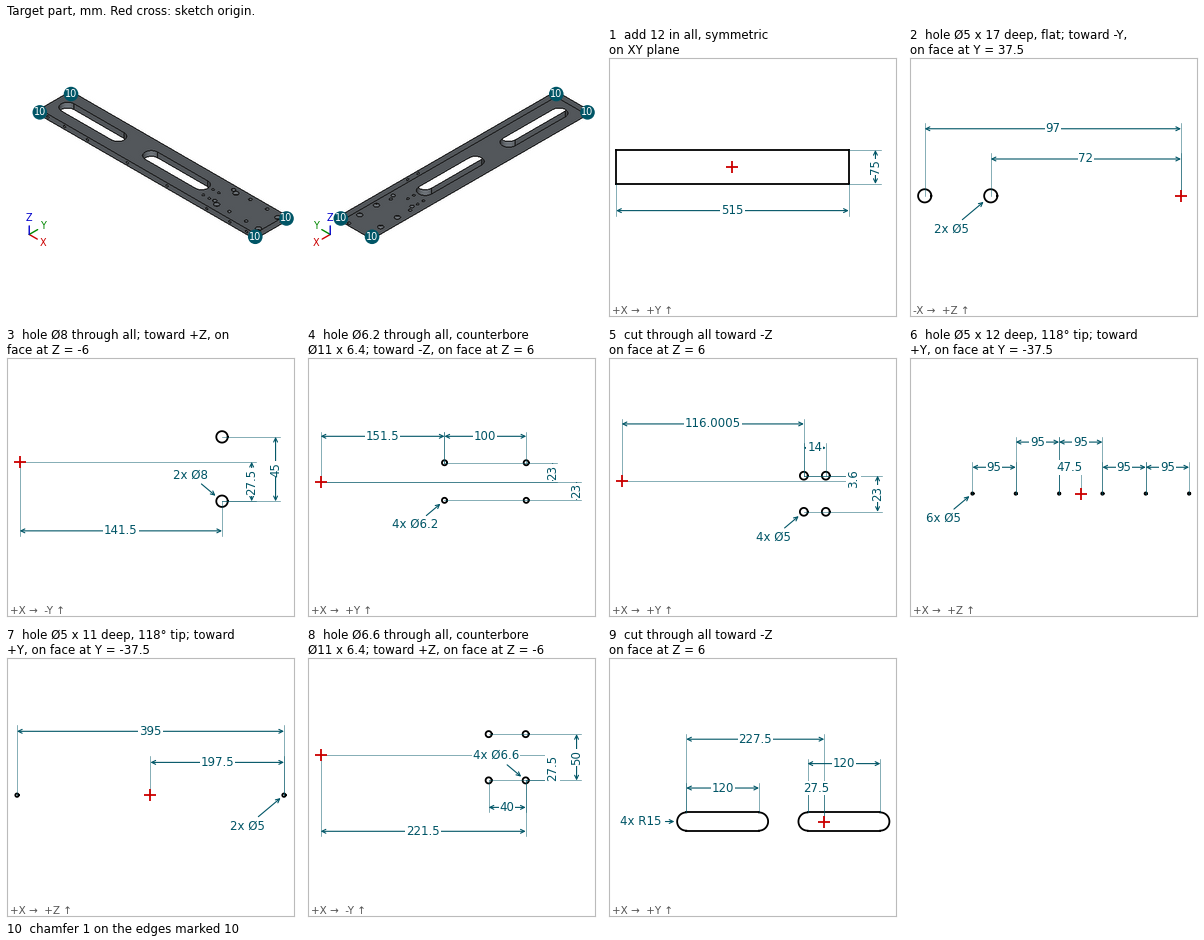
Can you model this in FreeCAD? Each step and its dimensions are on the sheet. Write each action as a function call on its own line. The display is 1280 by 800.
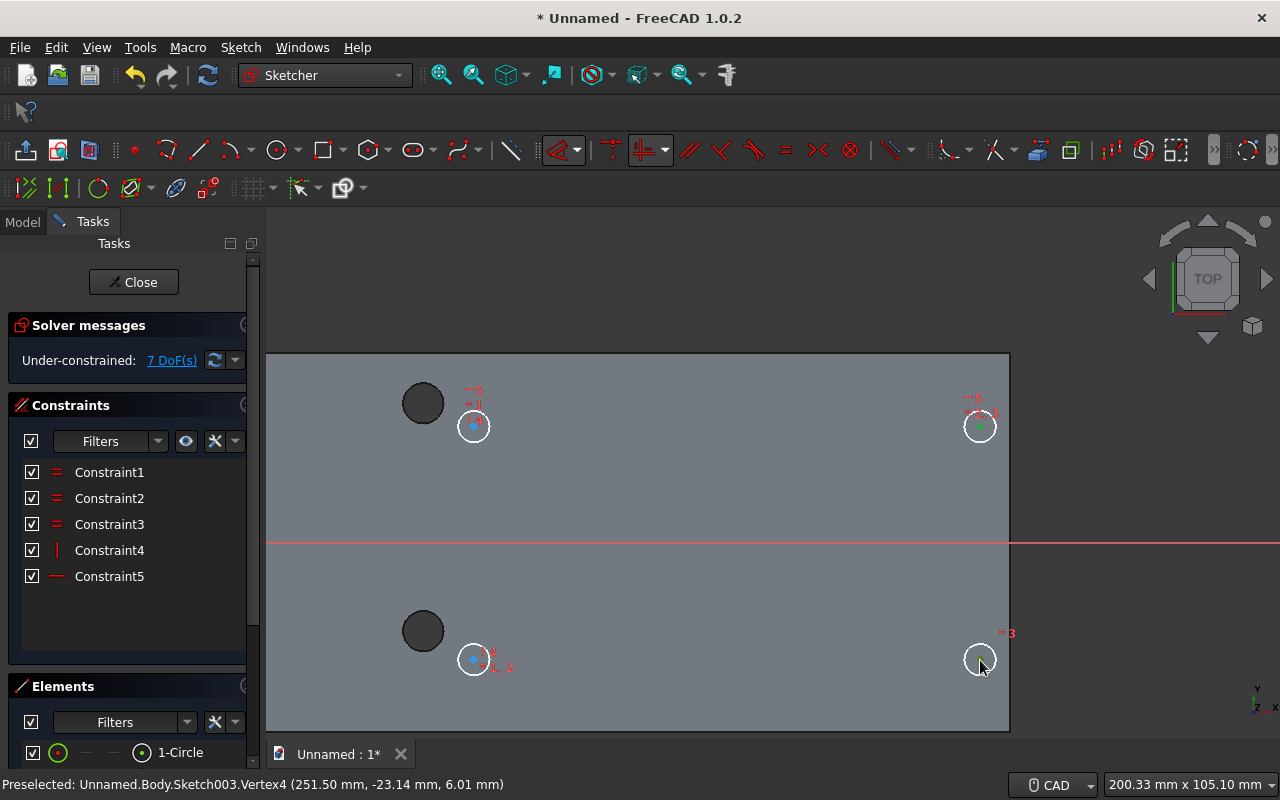
key(v)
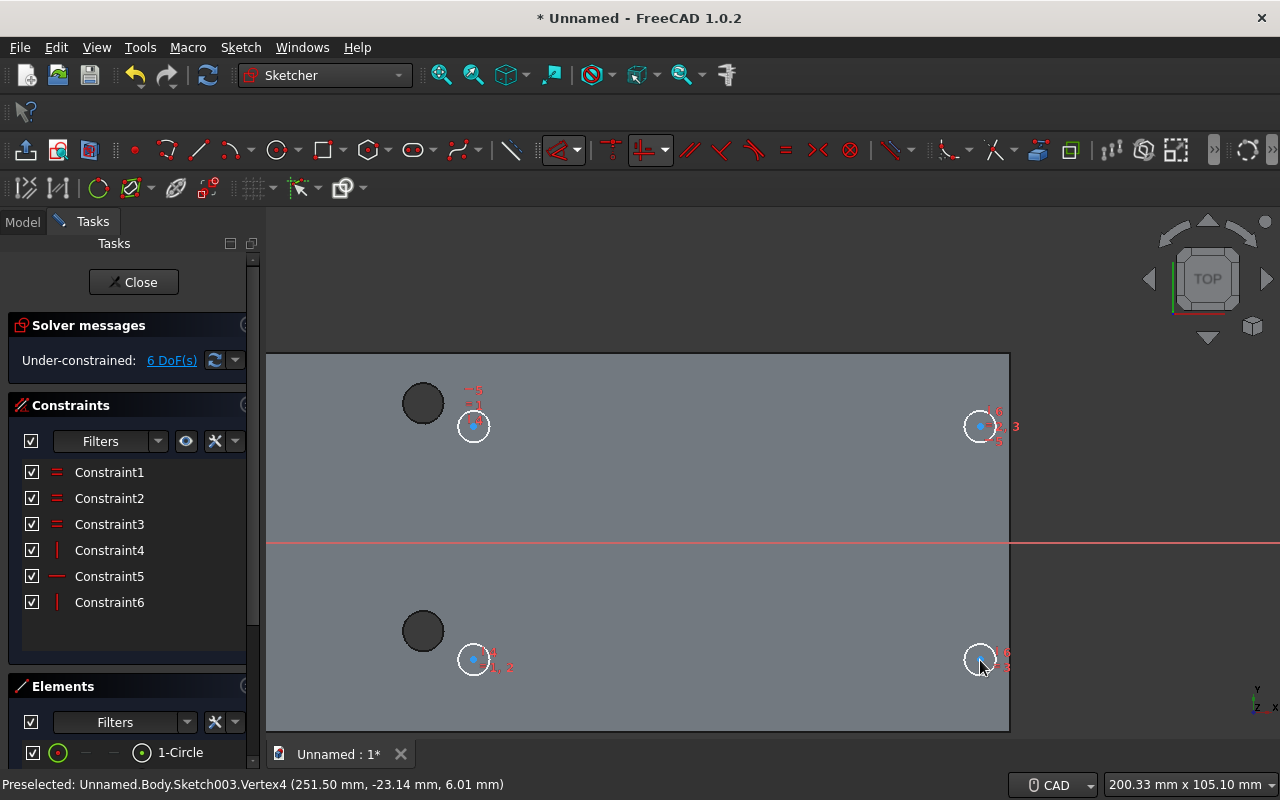
click(474, 660)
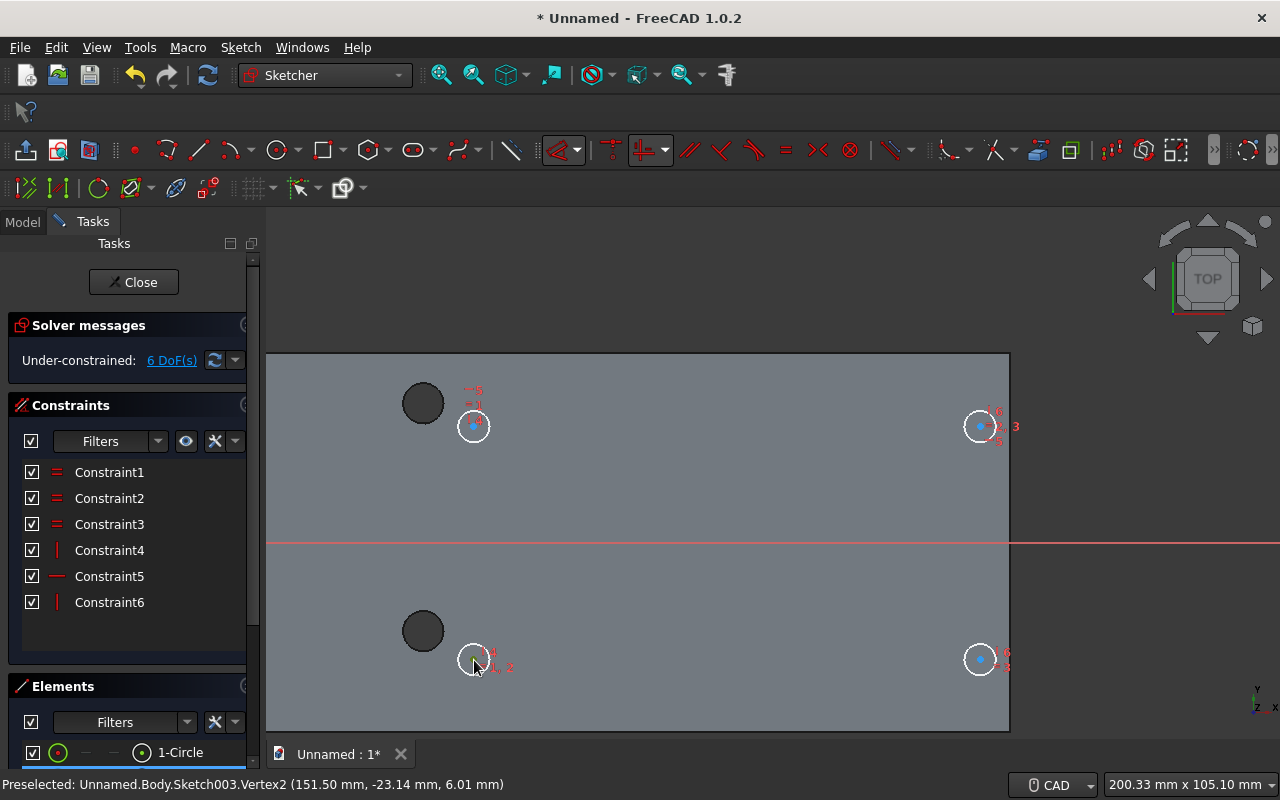
click(980, 660)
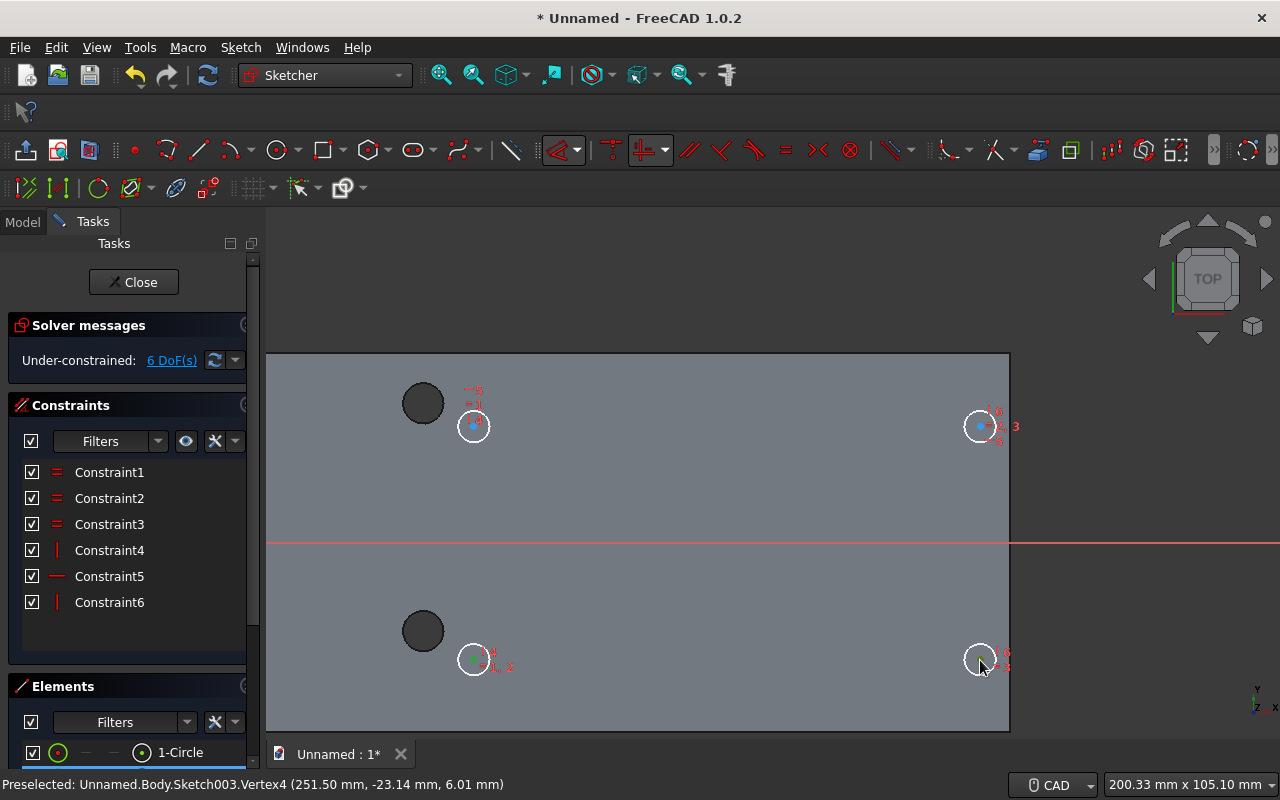
key(h)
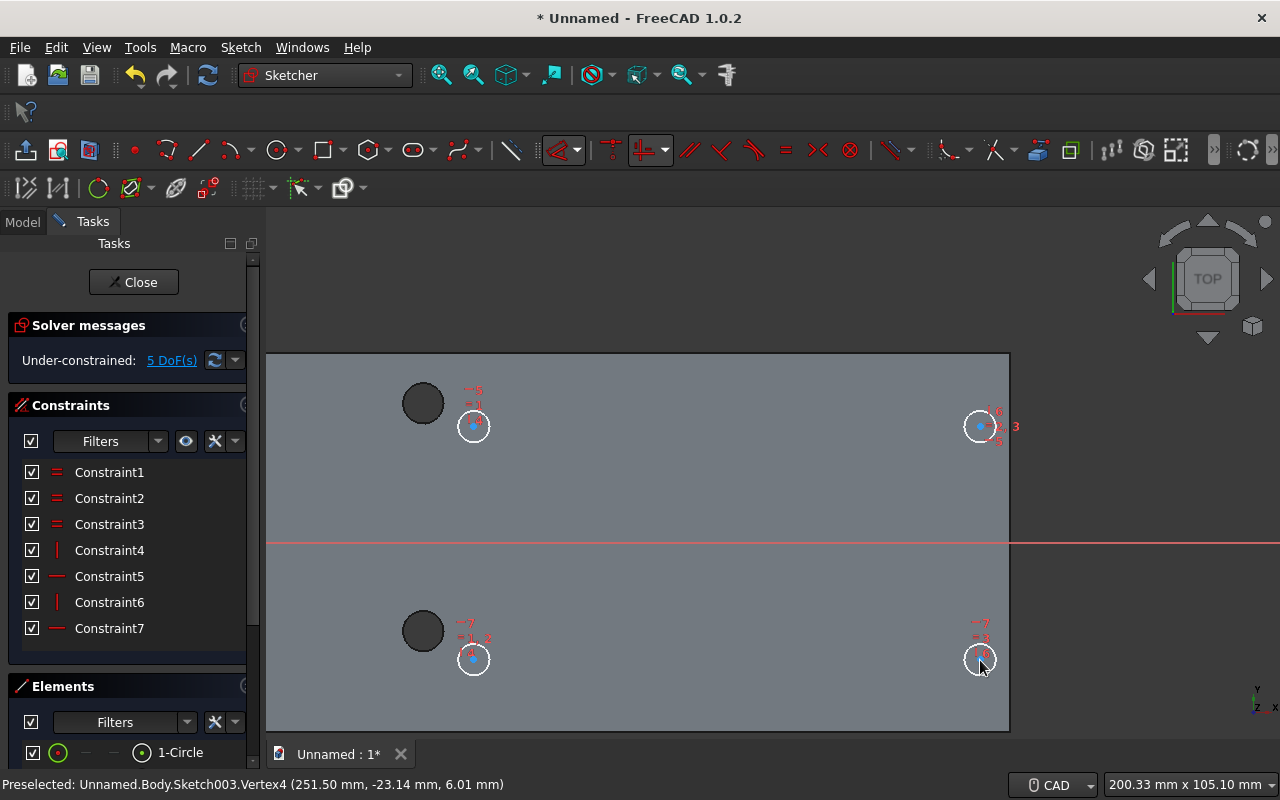
key(d)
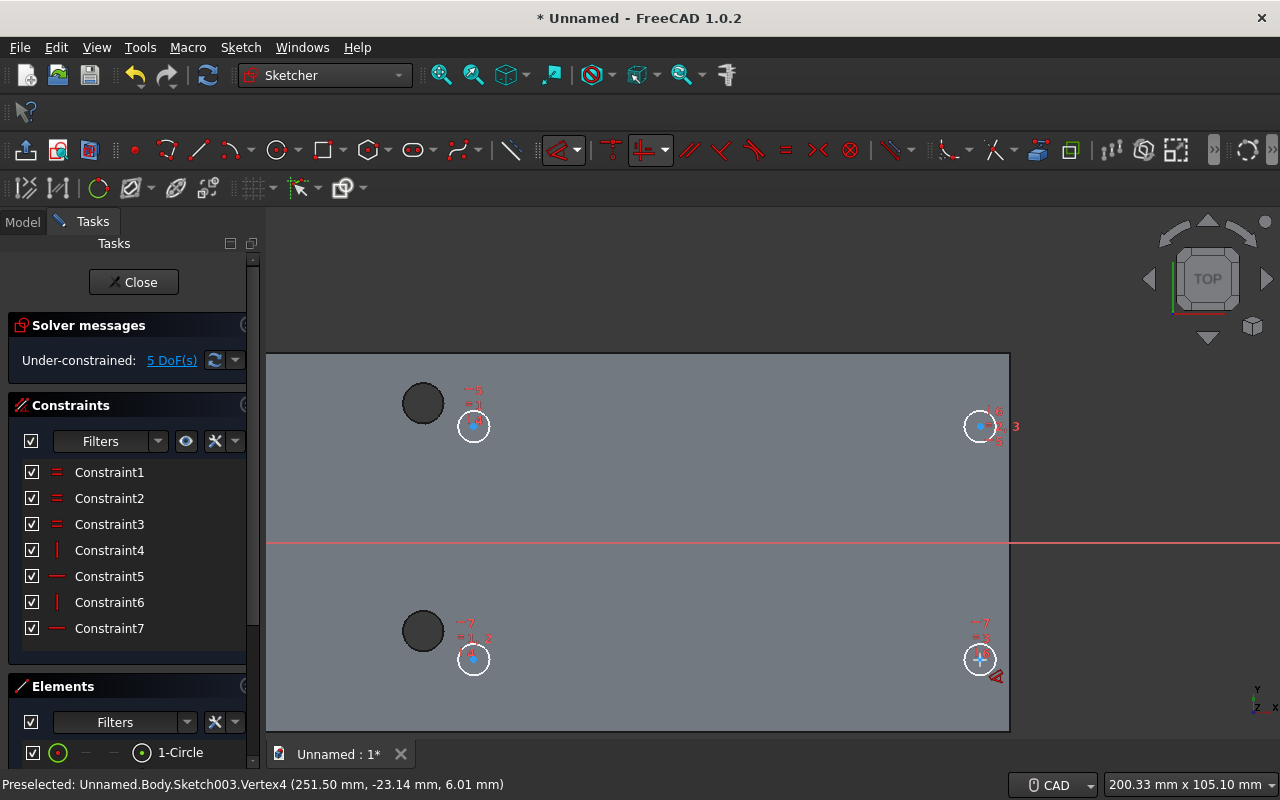
scroll(485, 416, up, 2)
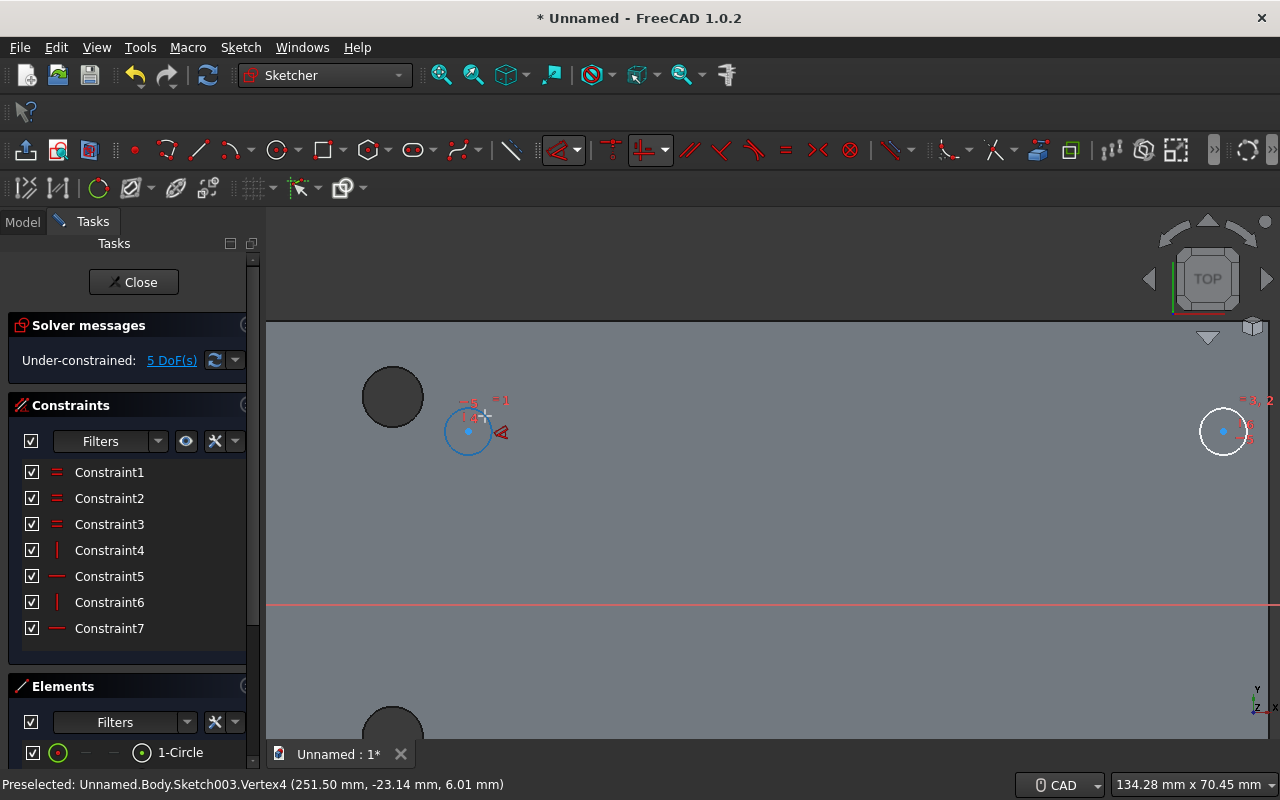
click(485, 415)
click(508, 392)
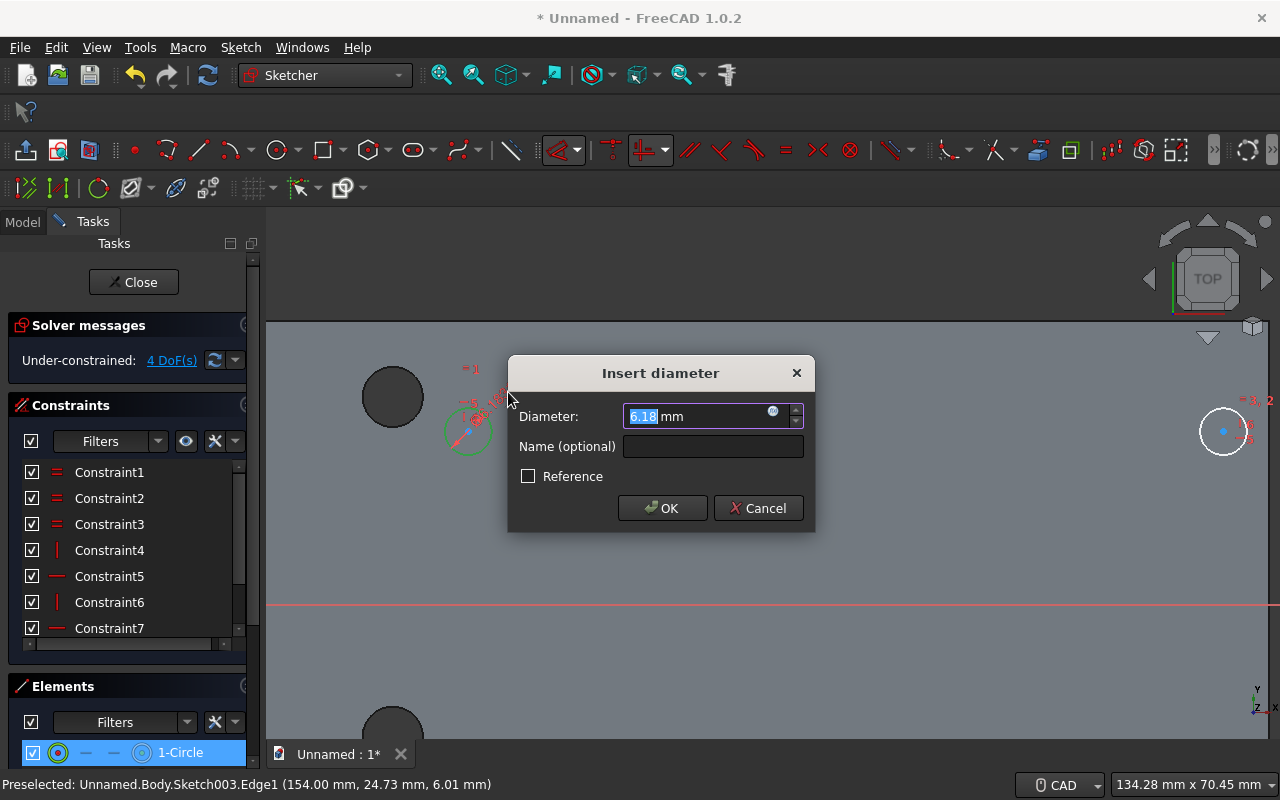
text(6.2)
key(Return)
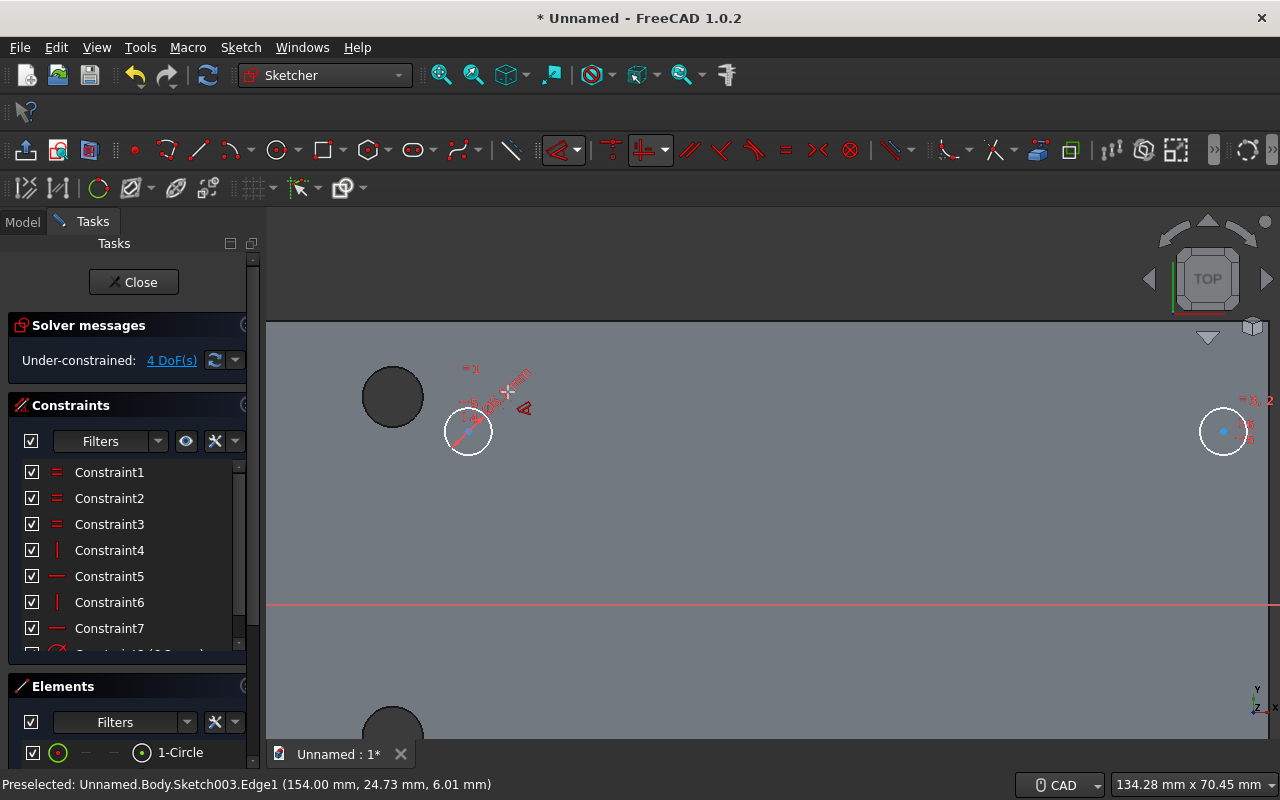
click(468, 432)
click(502, 518)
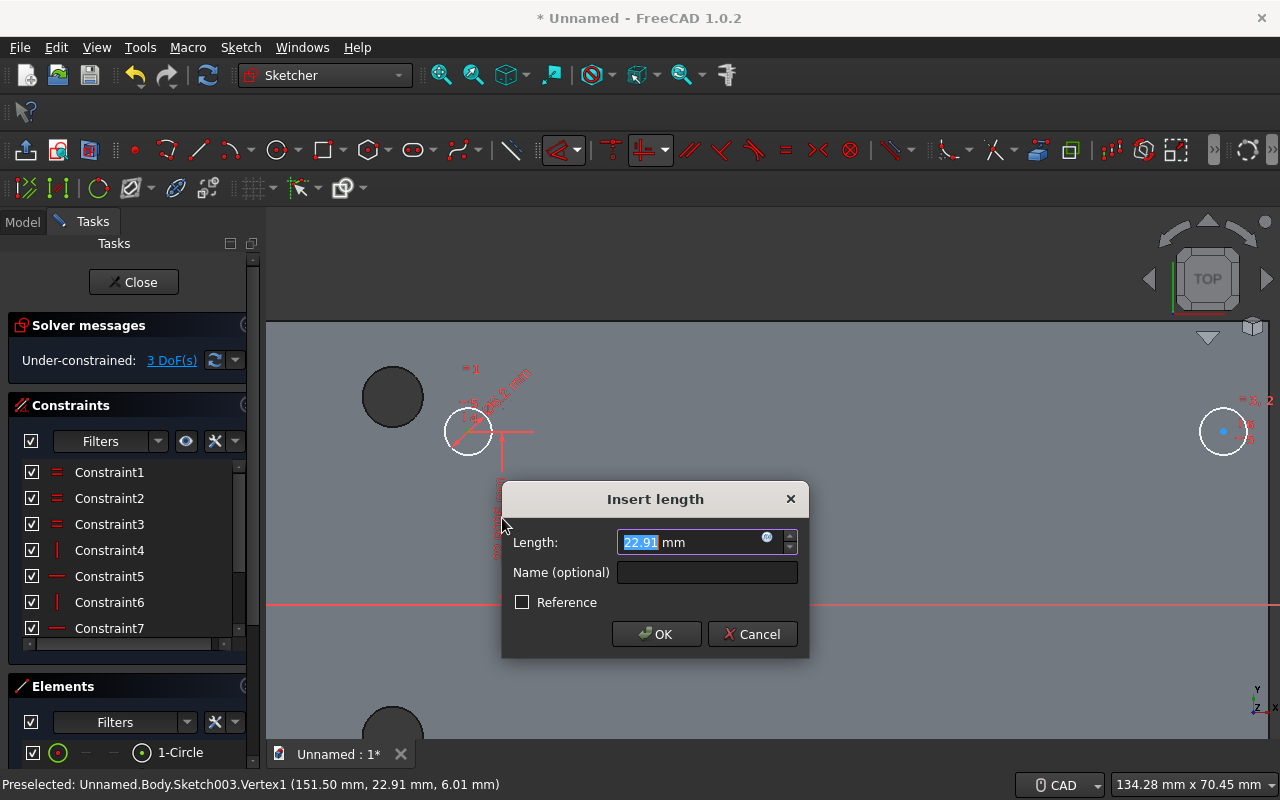
text(23)
key(Return)